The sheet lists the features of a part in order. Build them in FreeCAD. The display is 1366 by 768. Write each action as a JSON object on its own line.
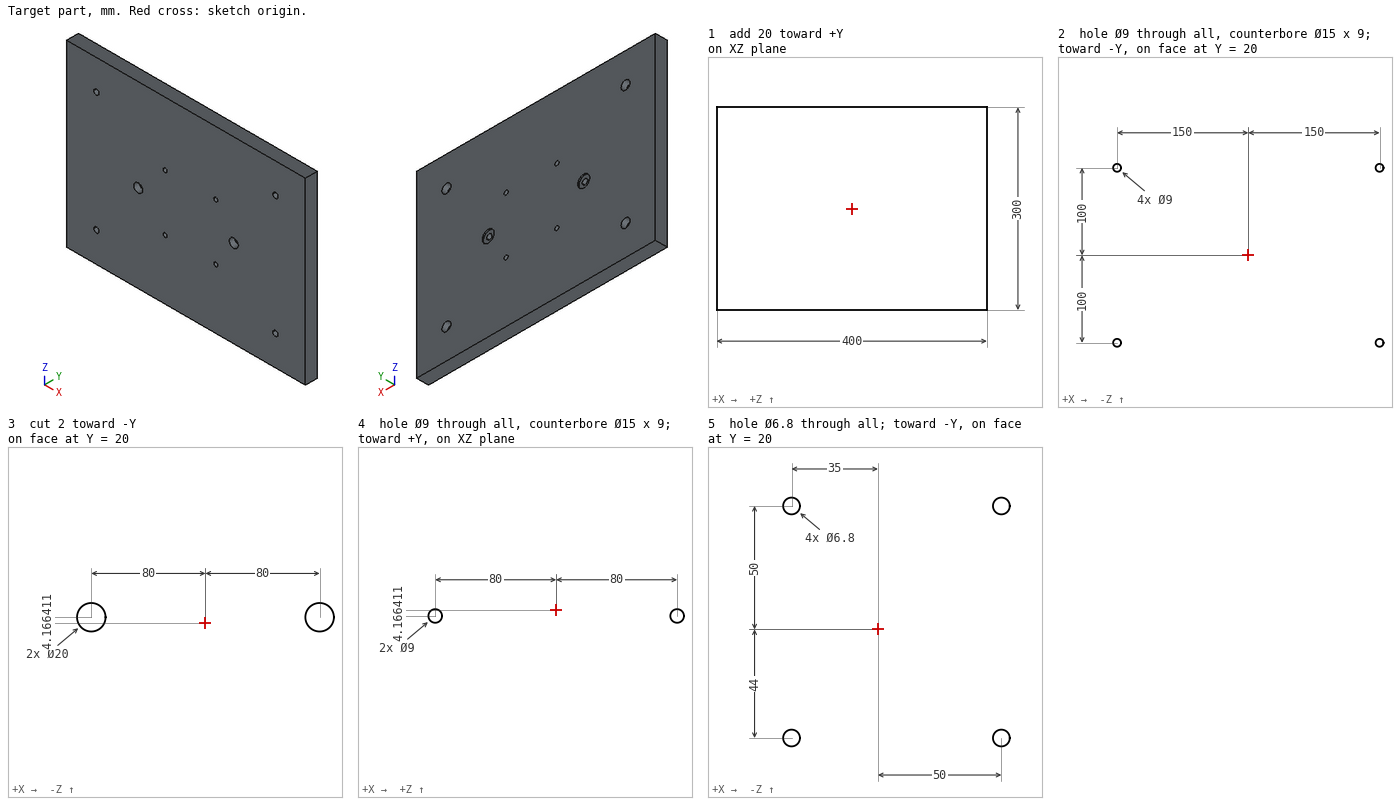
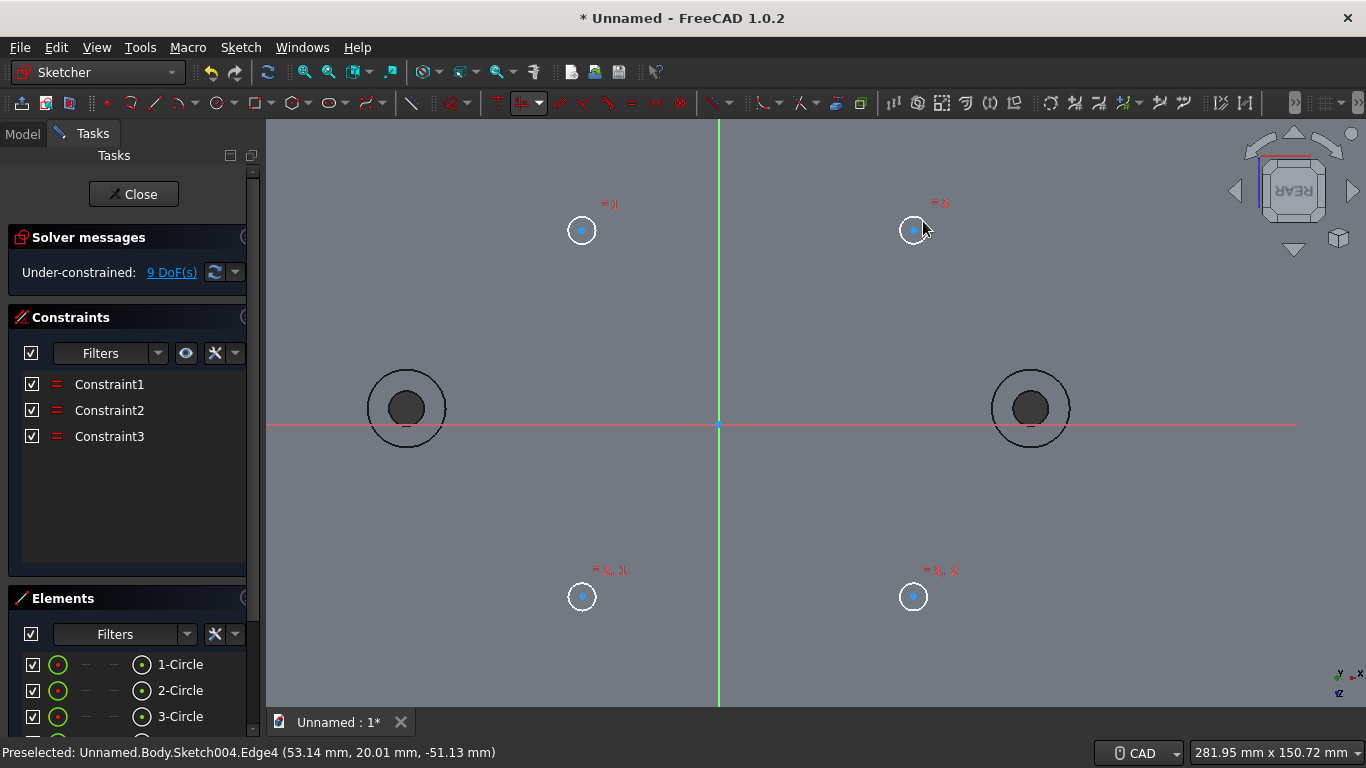
{"action": "left_click", "coordinate": [582, 231]}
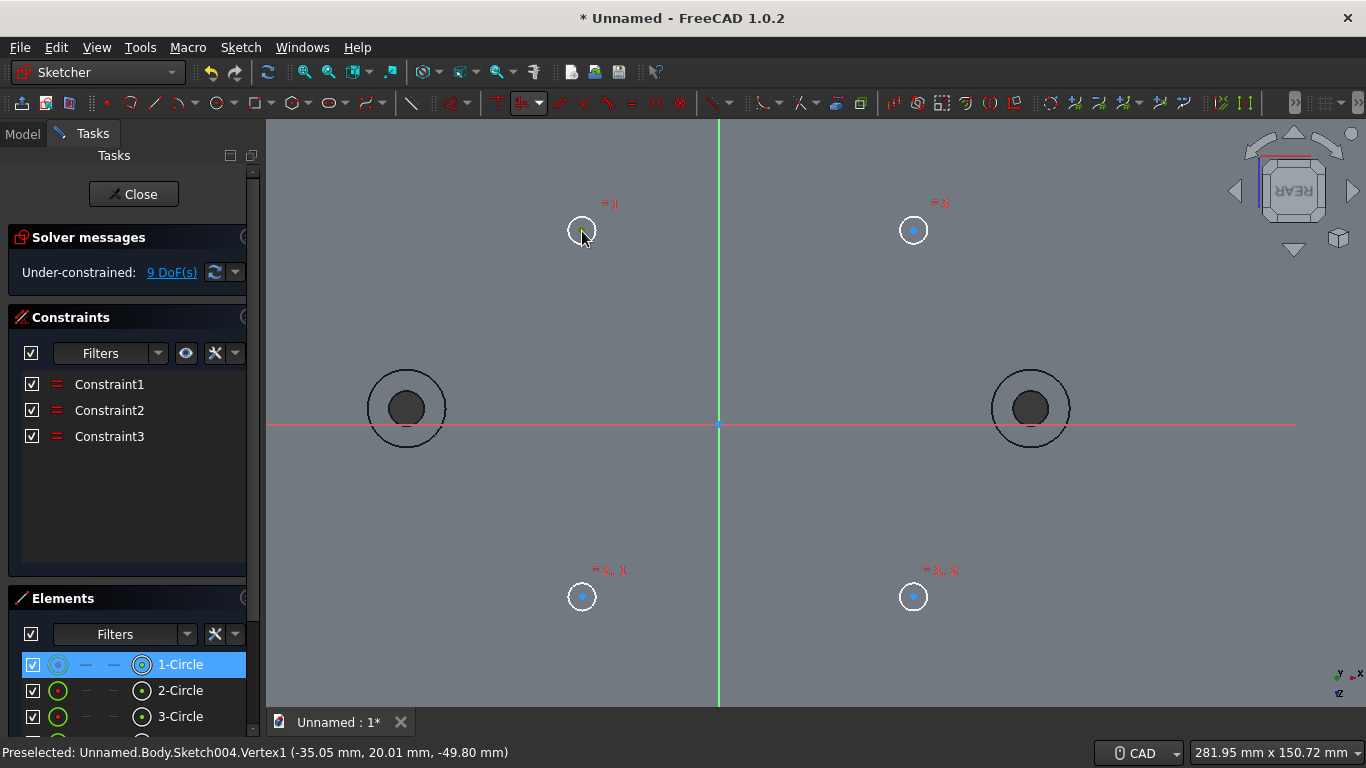
{"action": "left_click", "coordinate": [582, 597]}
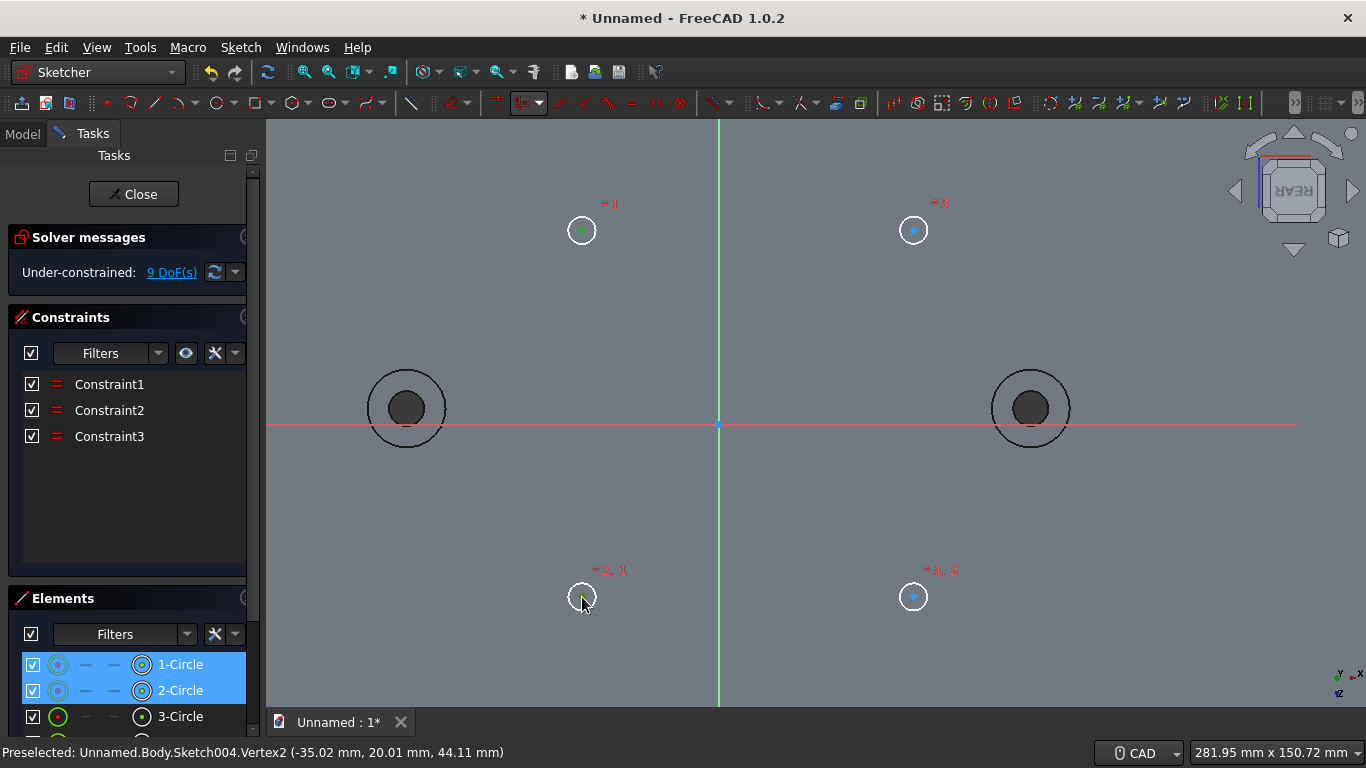
{"action": "left_click", "coordinate": [542, 104]}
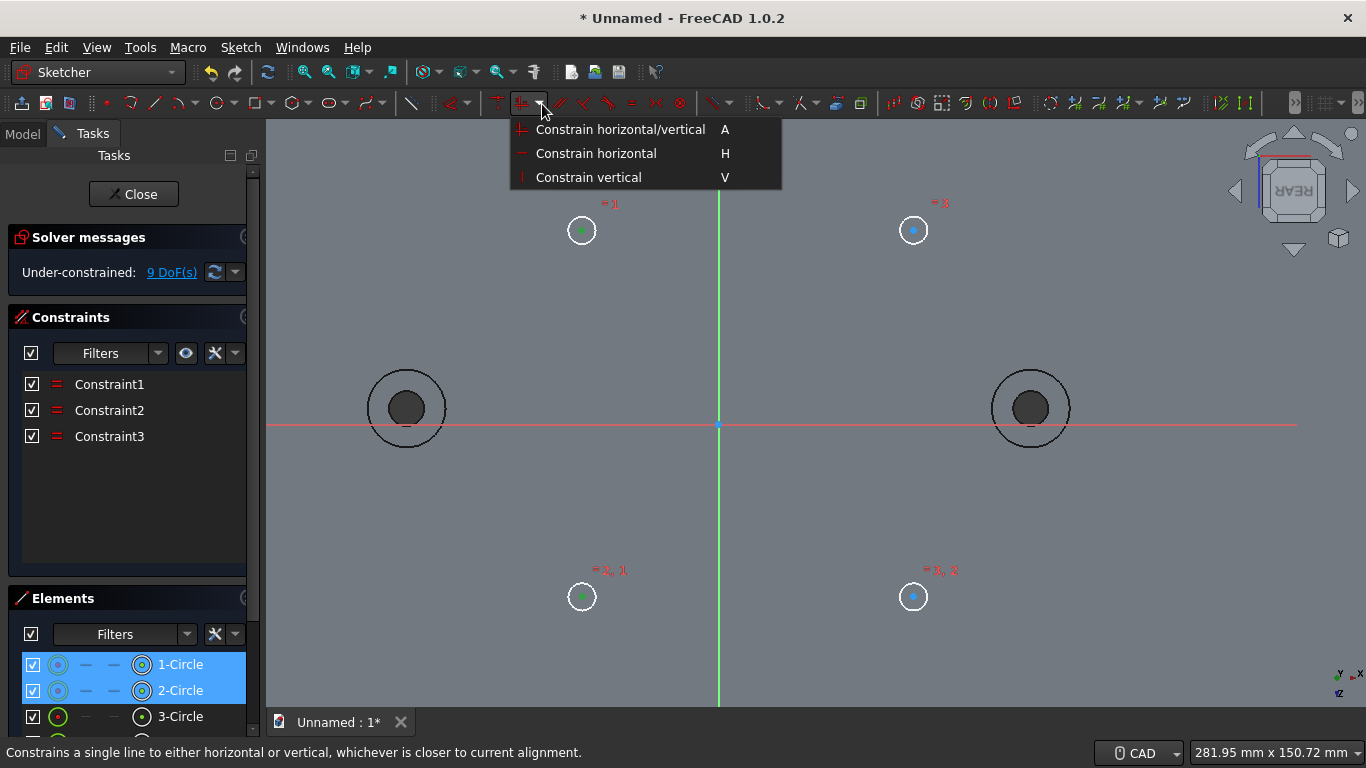
{"action": "left_click", "coordinate": [646, 177]}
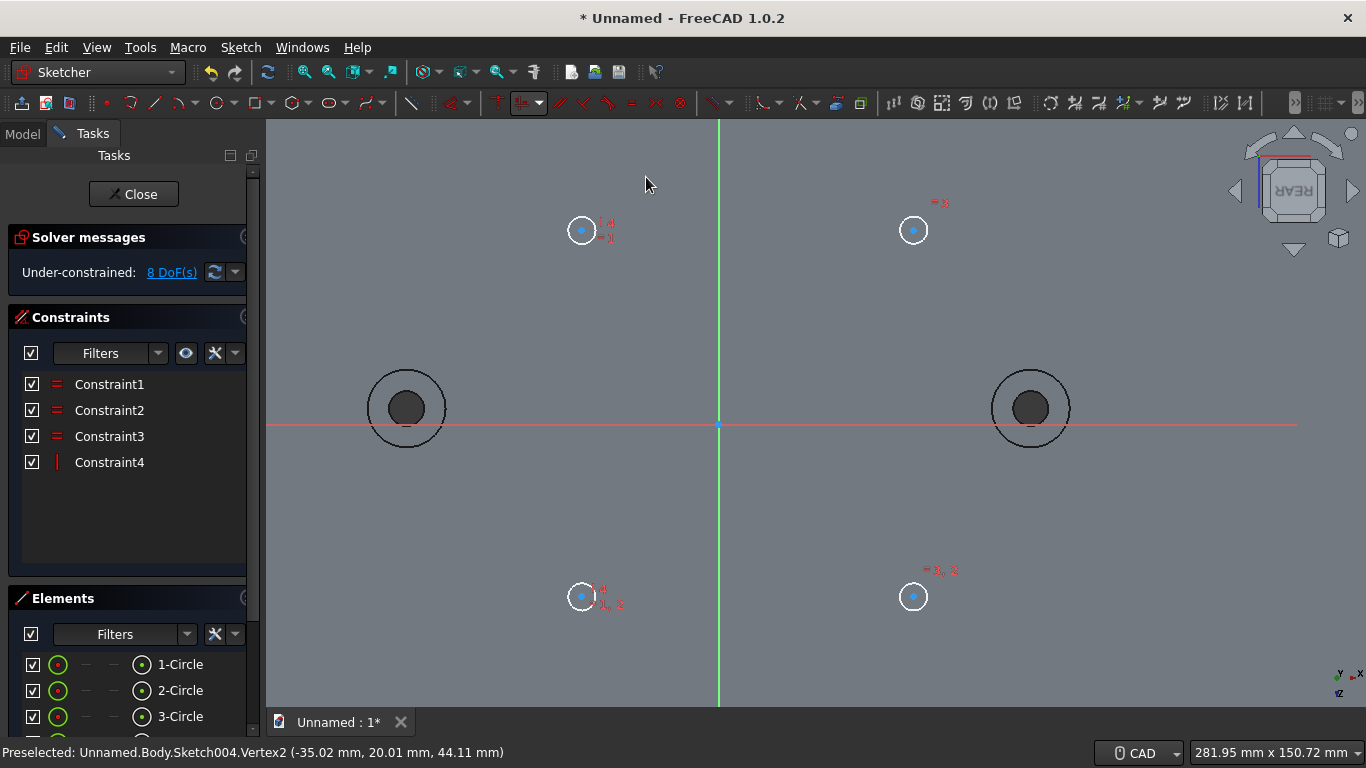
{"action": "left_click", "coordinate": [582, 597]}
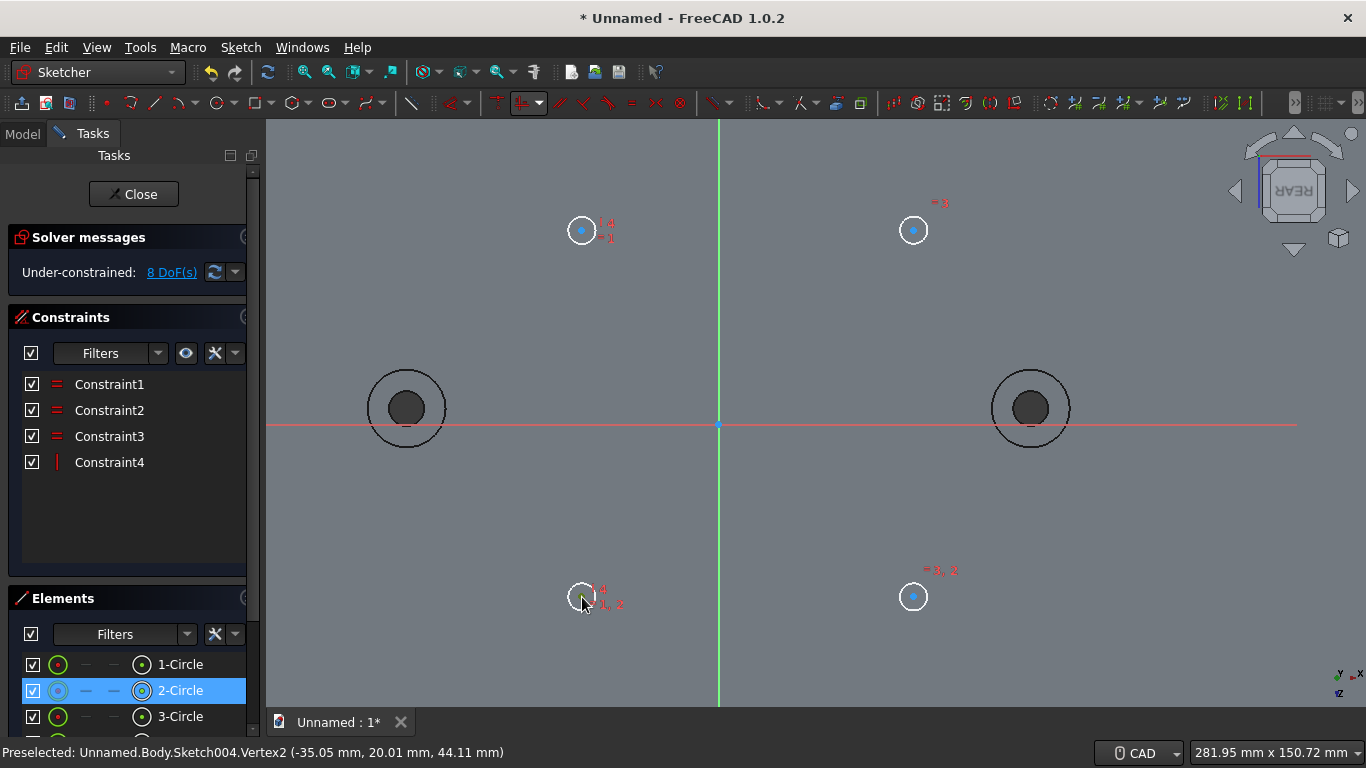
{"action": "left_click", "coordinate": [914, 597]}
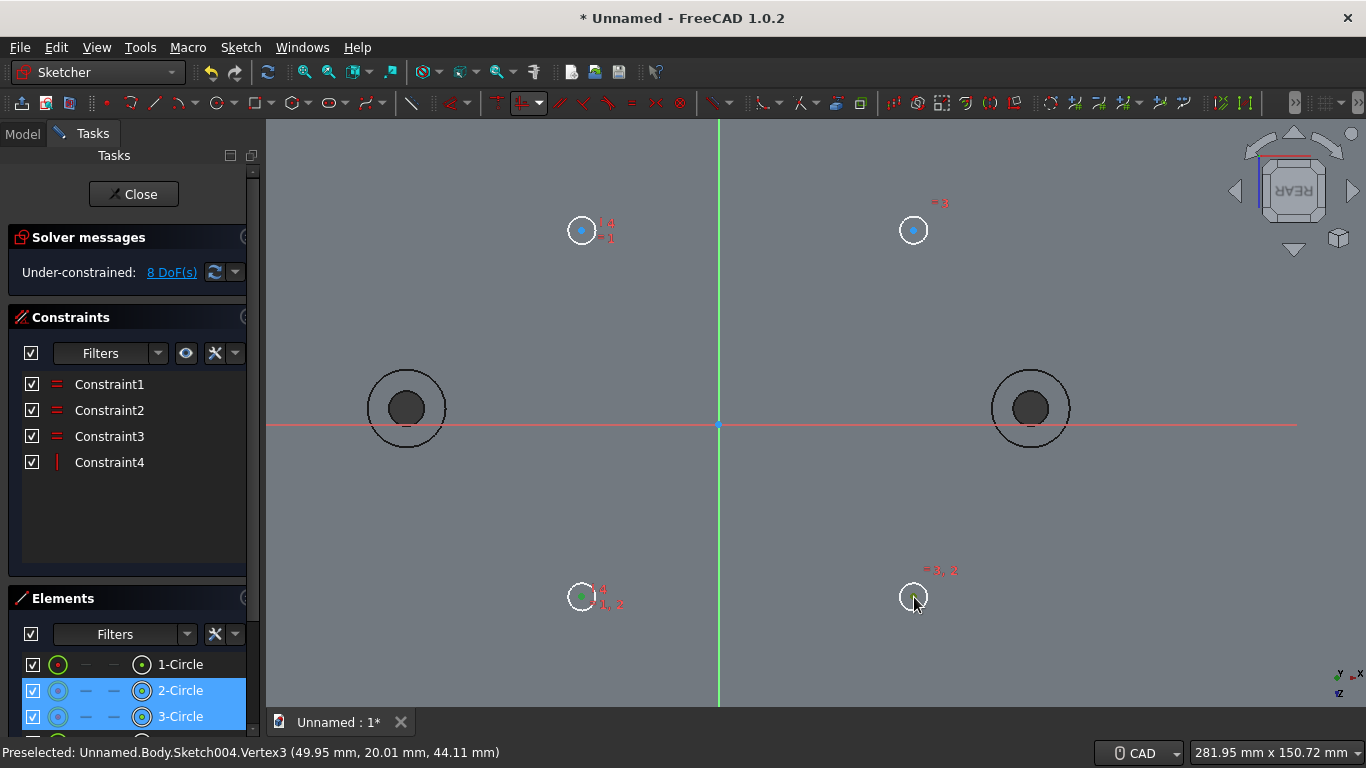
{"action": "key", "text": "h"}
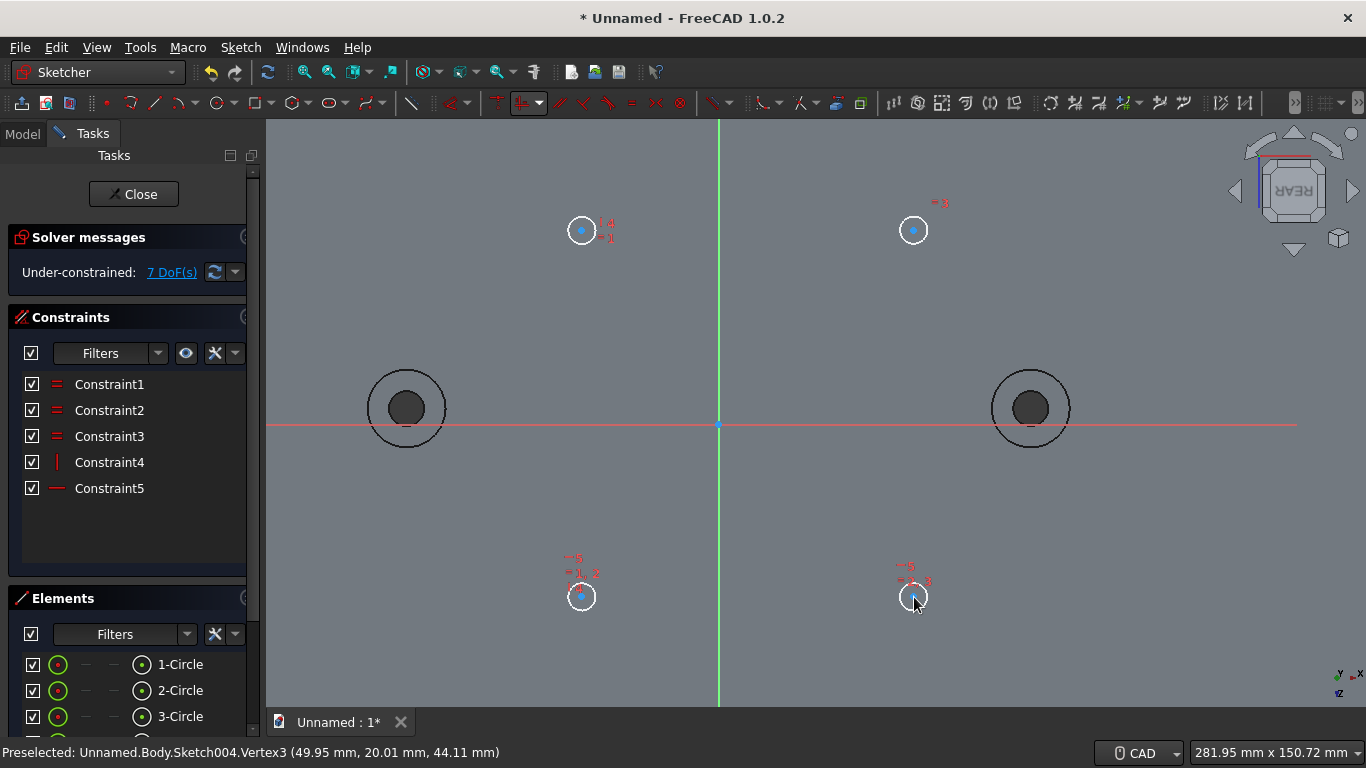
{"action": "left_click", "coordinate": [914, 597]}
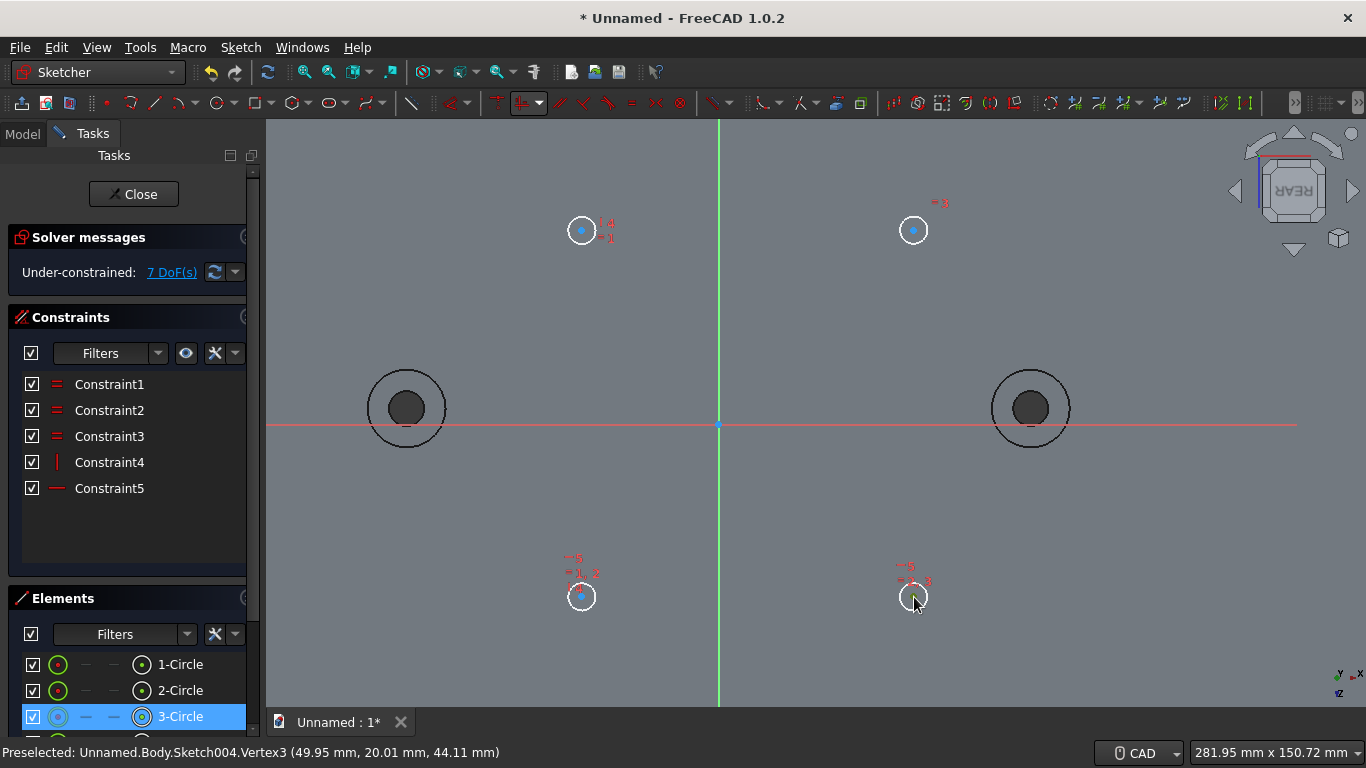
{"action": "left_click", "coordinate": [914, 230]}